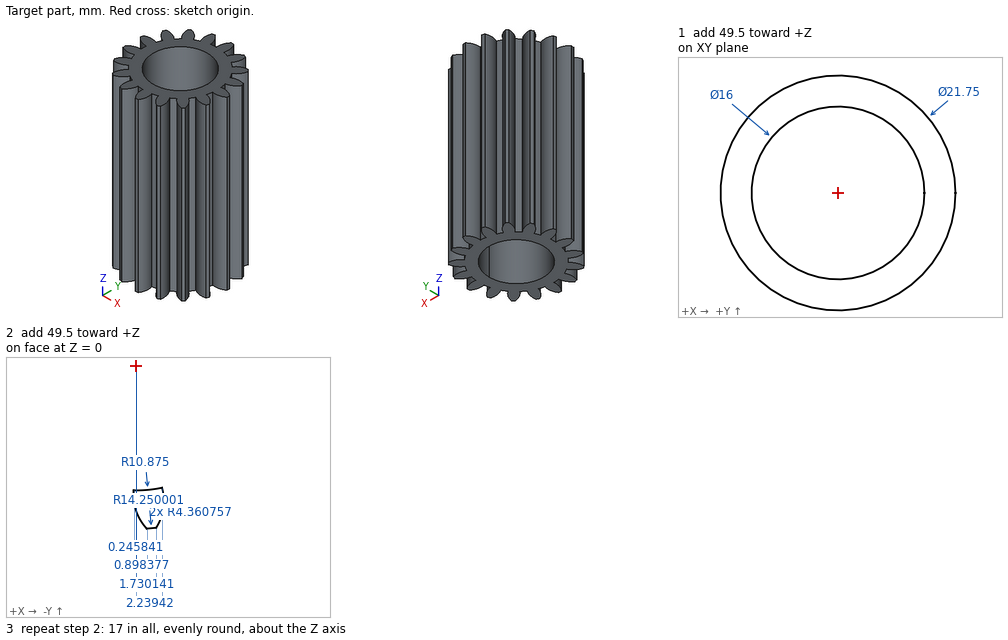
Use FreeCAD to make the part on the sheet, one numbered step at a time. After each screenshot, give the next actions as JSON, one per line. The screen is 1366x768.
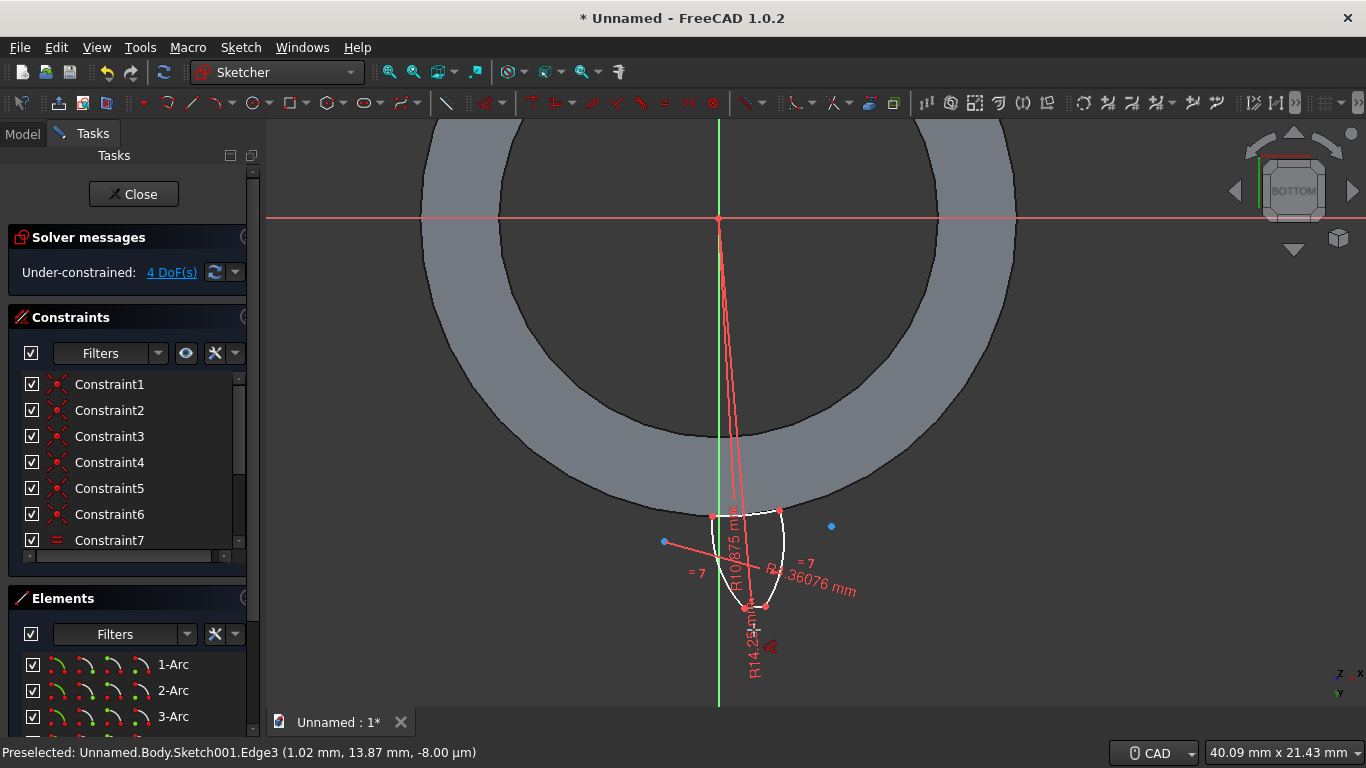
{"action": "left_click", "coordinate": [780, 510]}
{"action": "left_click", "coordinate": [749, 184]}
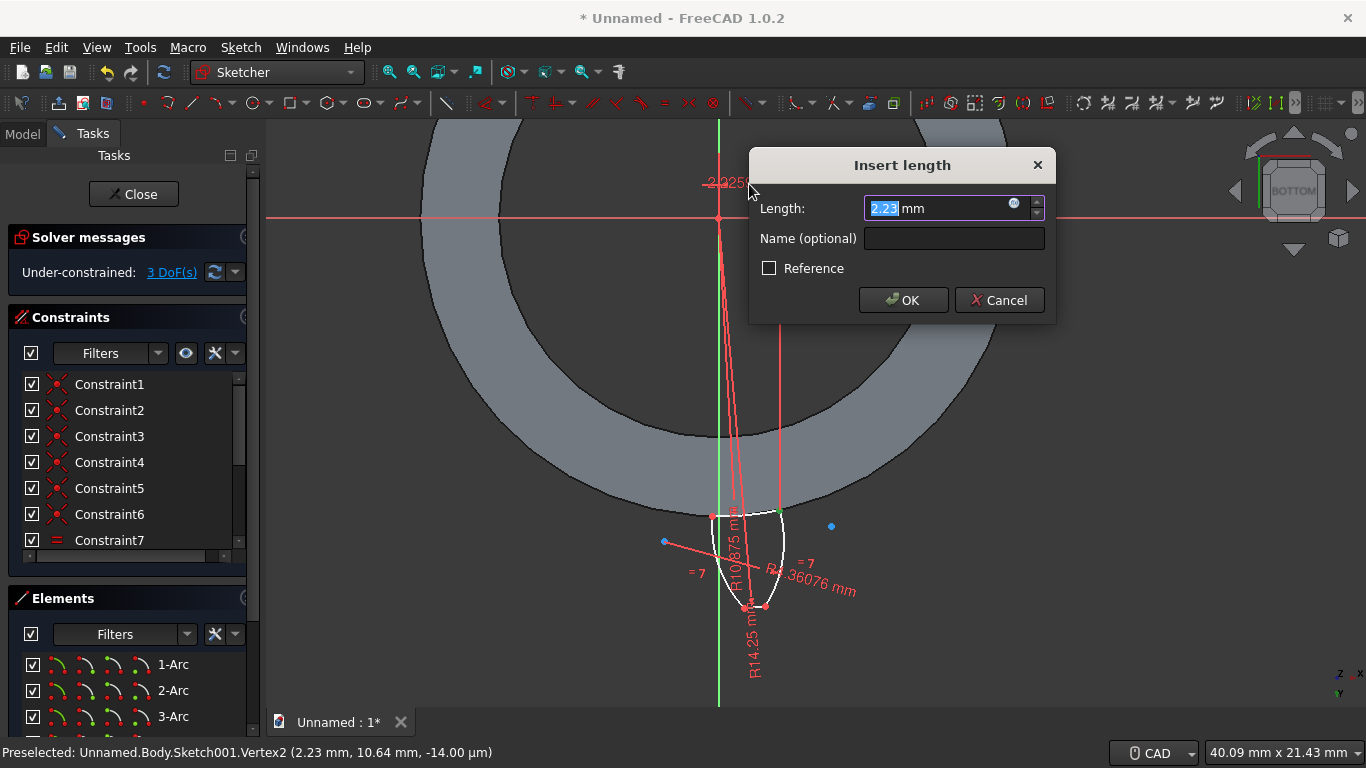
{"action": "type", "text": "2.23942"}
{"action": "key", "text": "Return"}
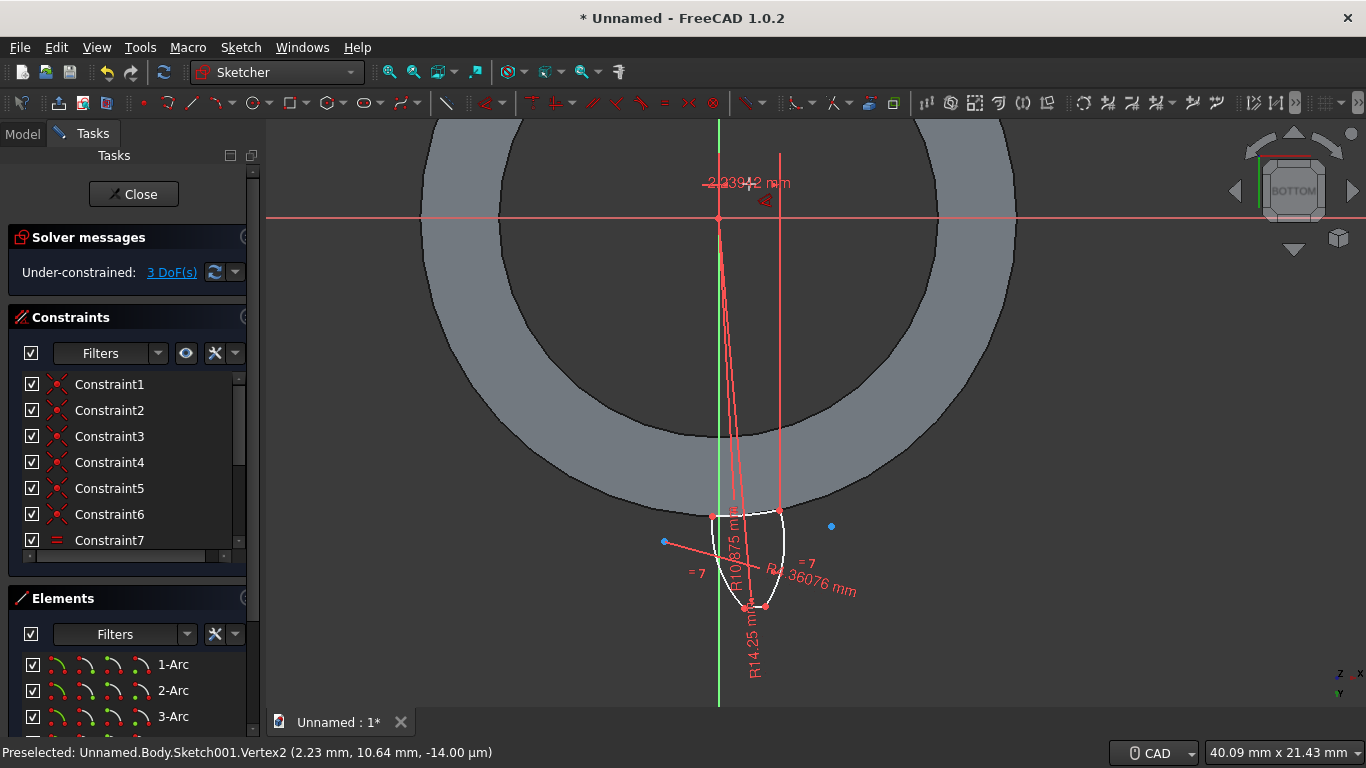
{"action": "scroll", "coordinate": [713, 516], "scroll_direction": "up", "scroll_amount": 9}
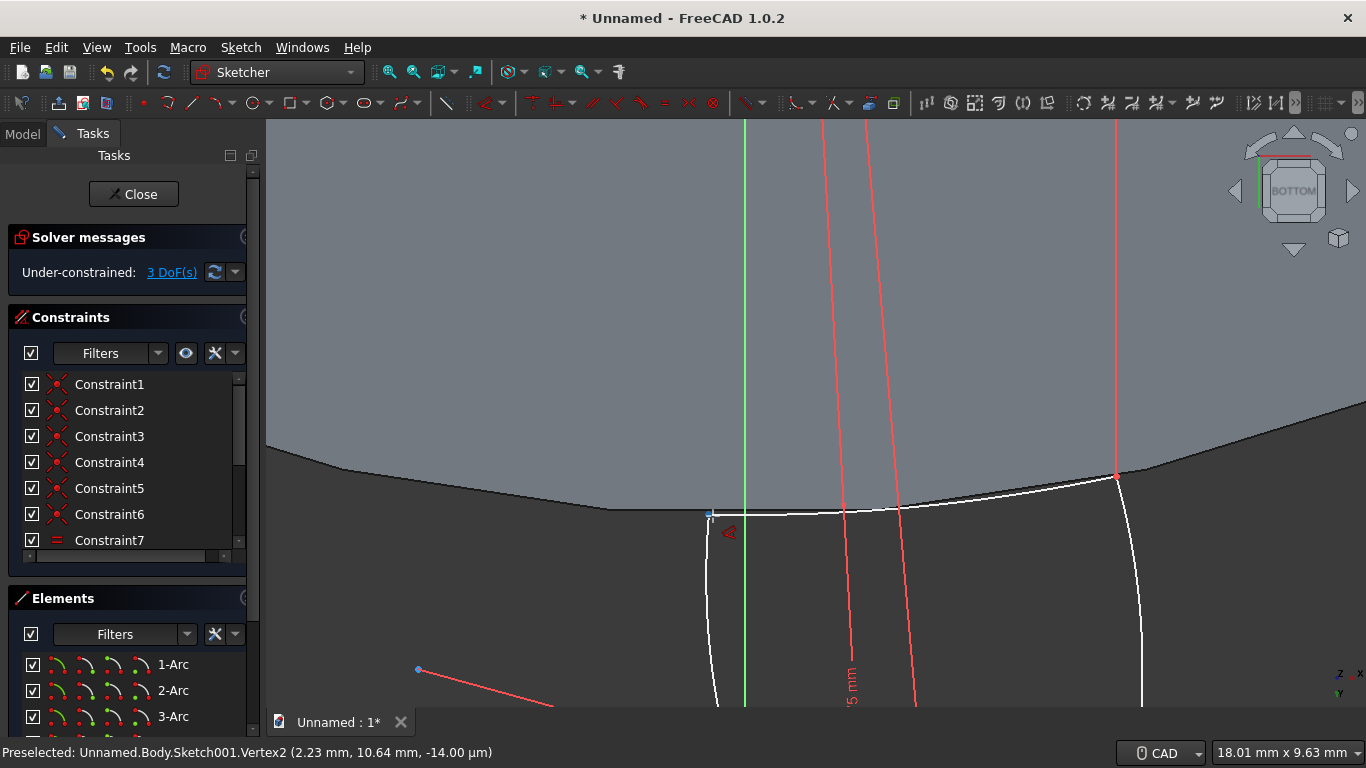
{"action": "left_click", "coordinate": [709, 515]}
{"action": "left_click", "coordinate": [727, 549]}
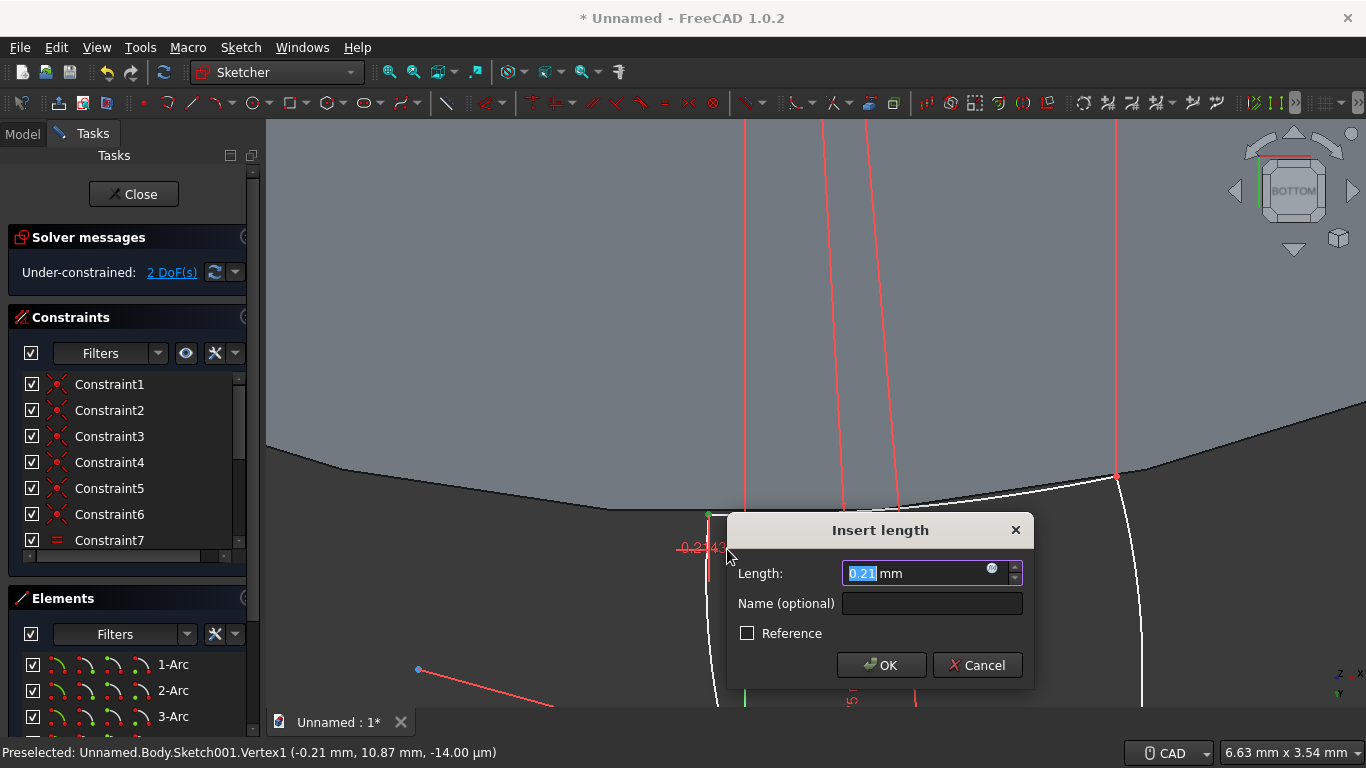
{"action": "type", "text": "0.245841"}
{"action": "key", "text": "Return"}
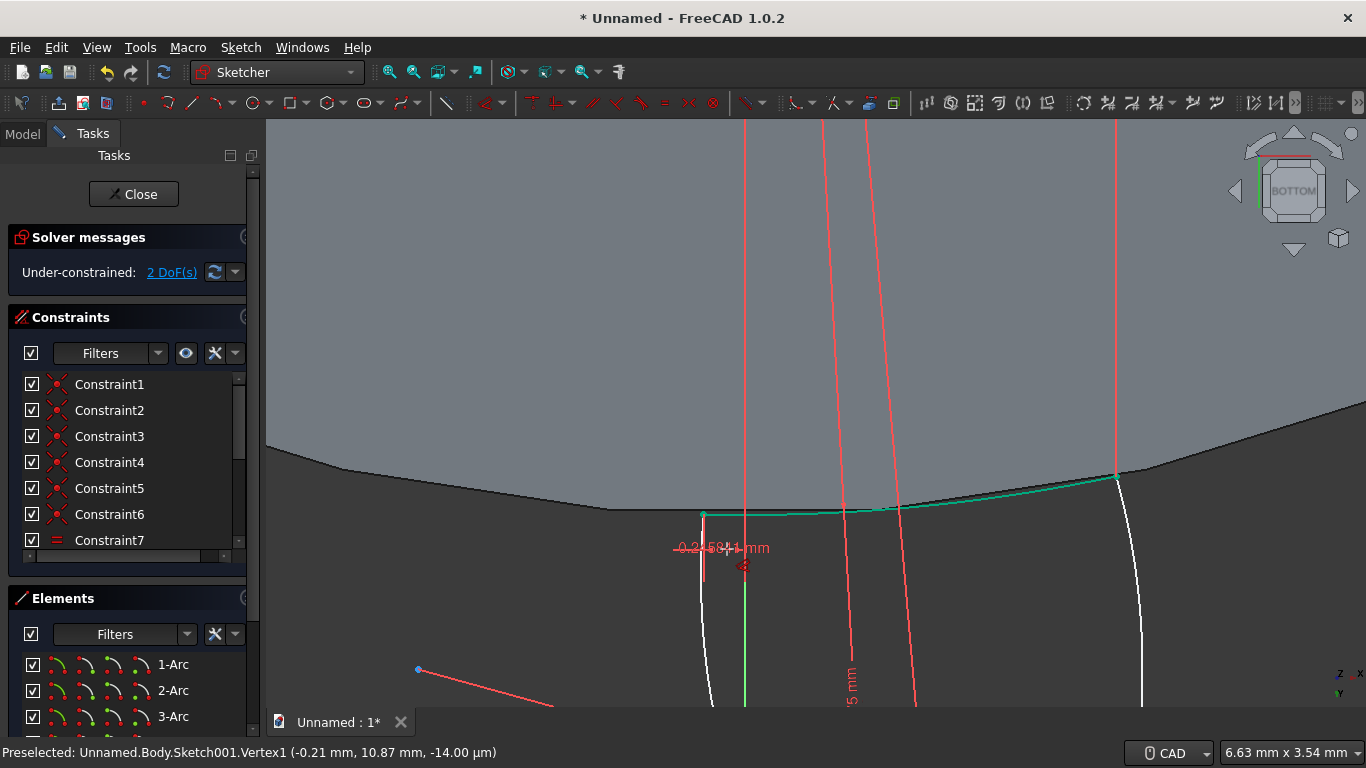
{"action": "scroll", "coordinate": [538, 147], "scroll_direction": "down", "scroll_amount": 3}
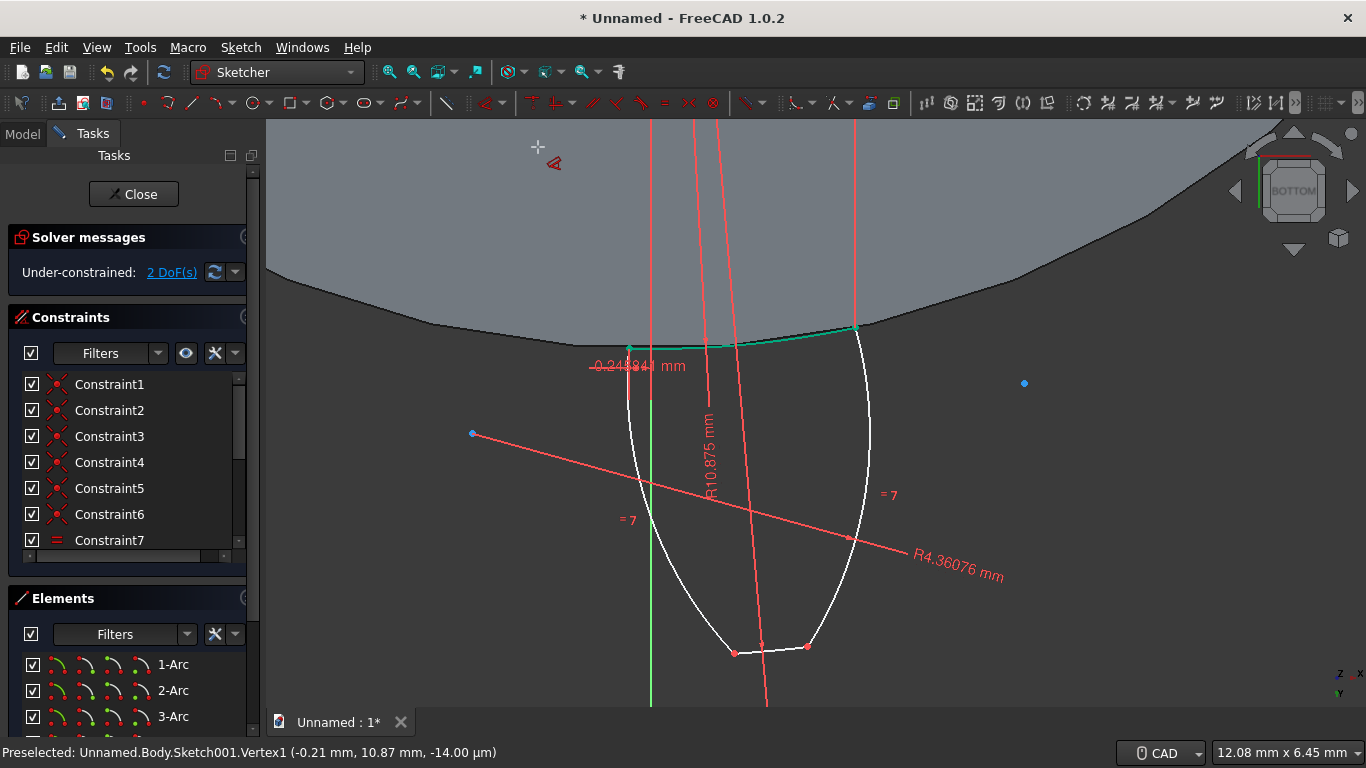
{"action": "left_click", "coordinate": [808, 647]}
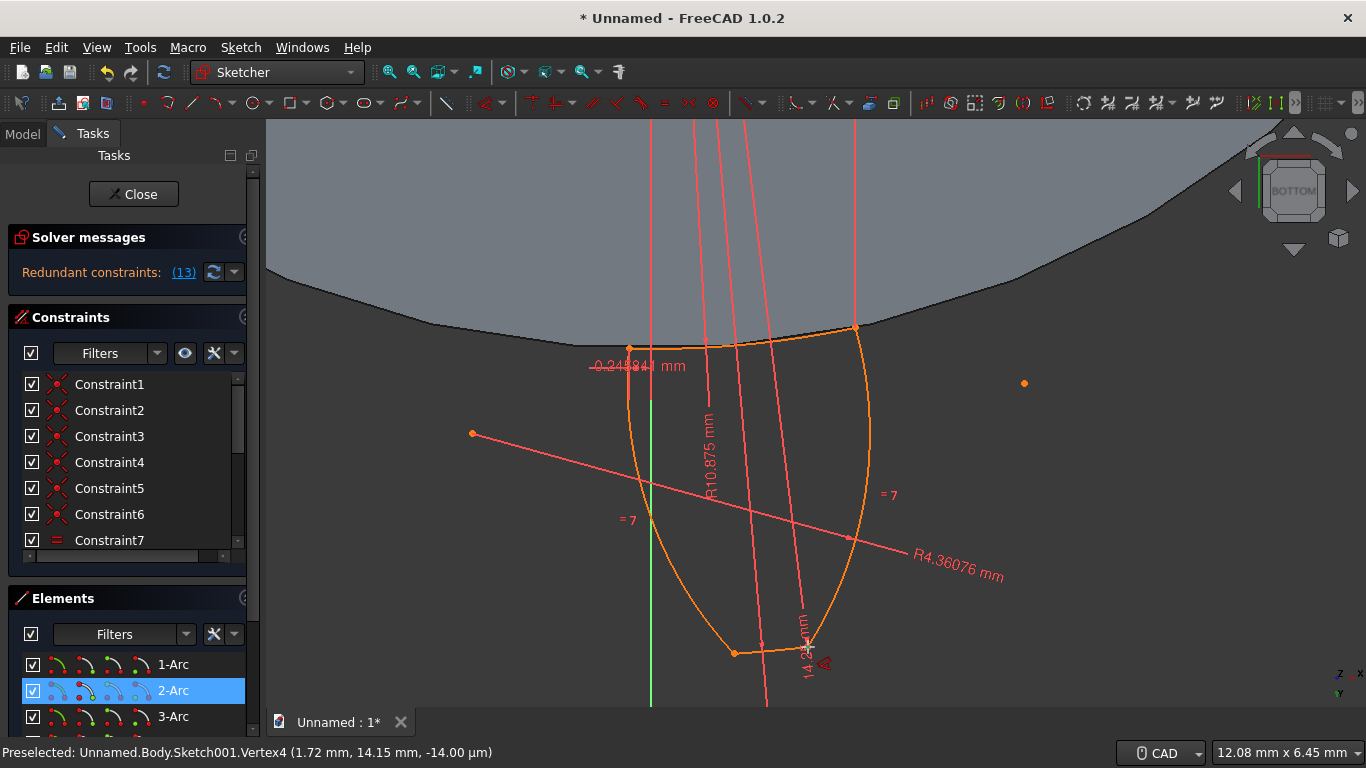
{"action": "key", "text": "Escape"}
{"action": "key", "text": "Escape"}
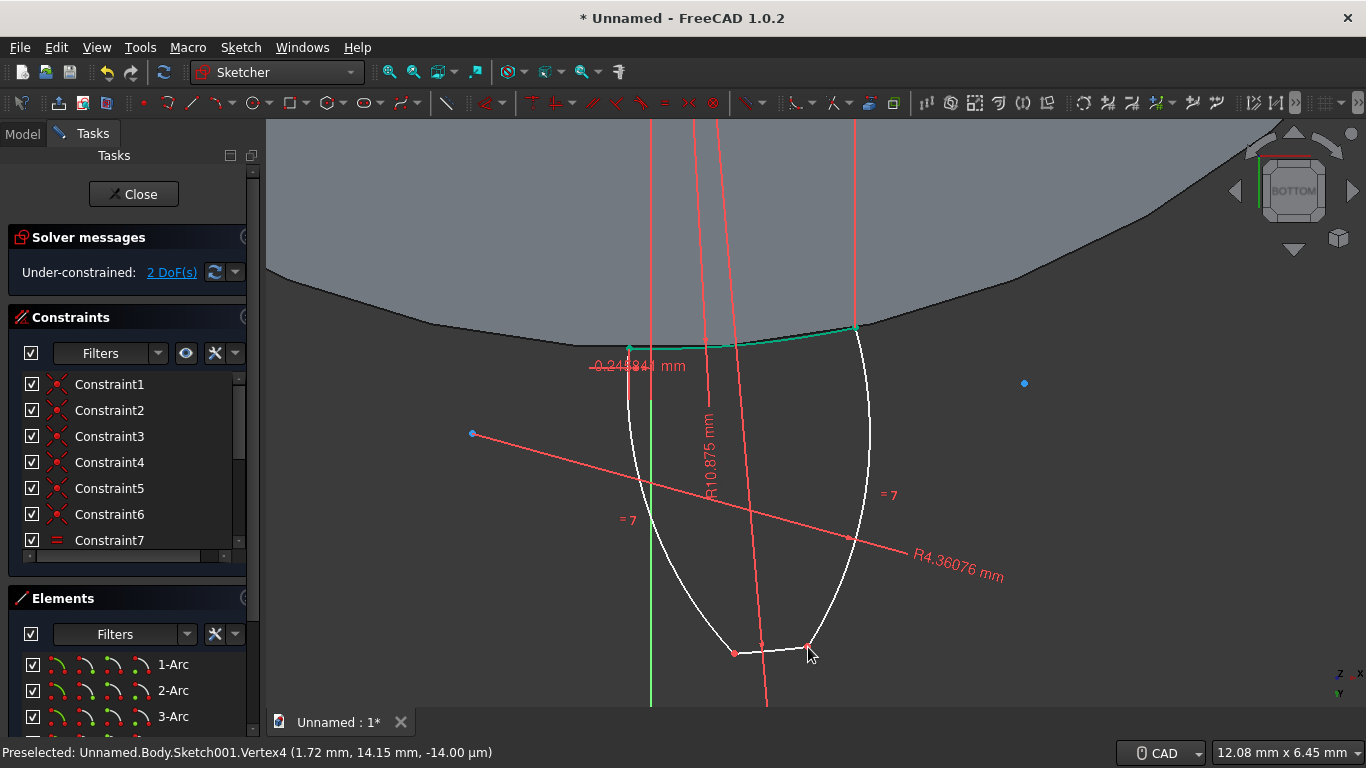
{"action": "left_click", "coordinate": [808, 647]}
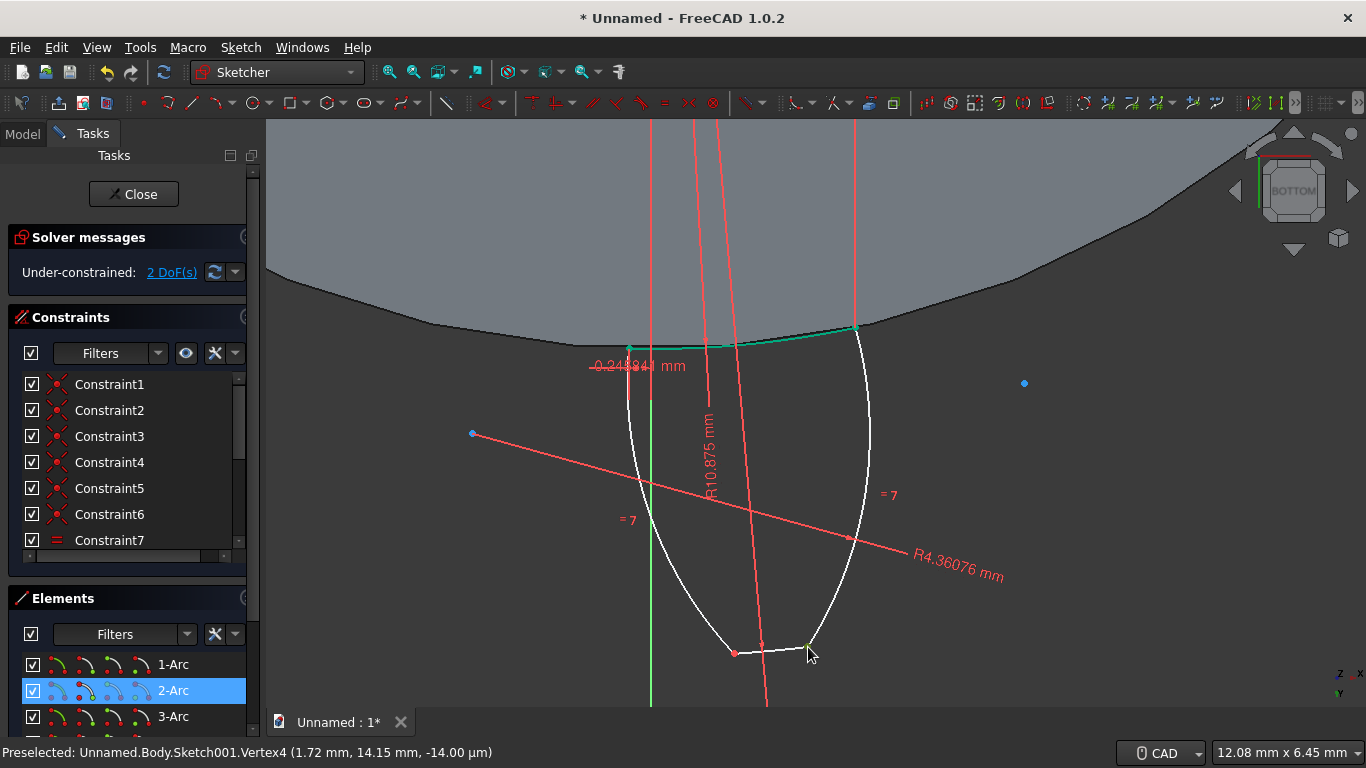
{"action": "left_click", "coordinate": [504, 104]}